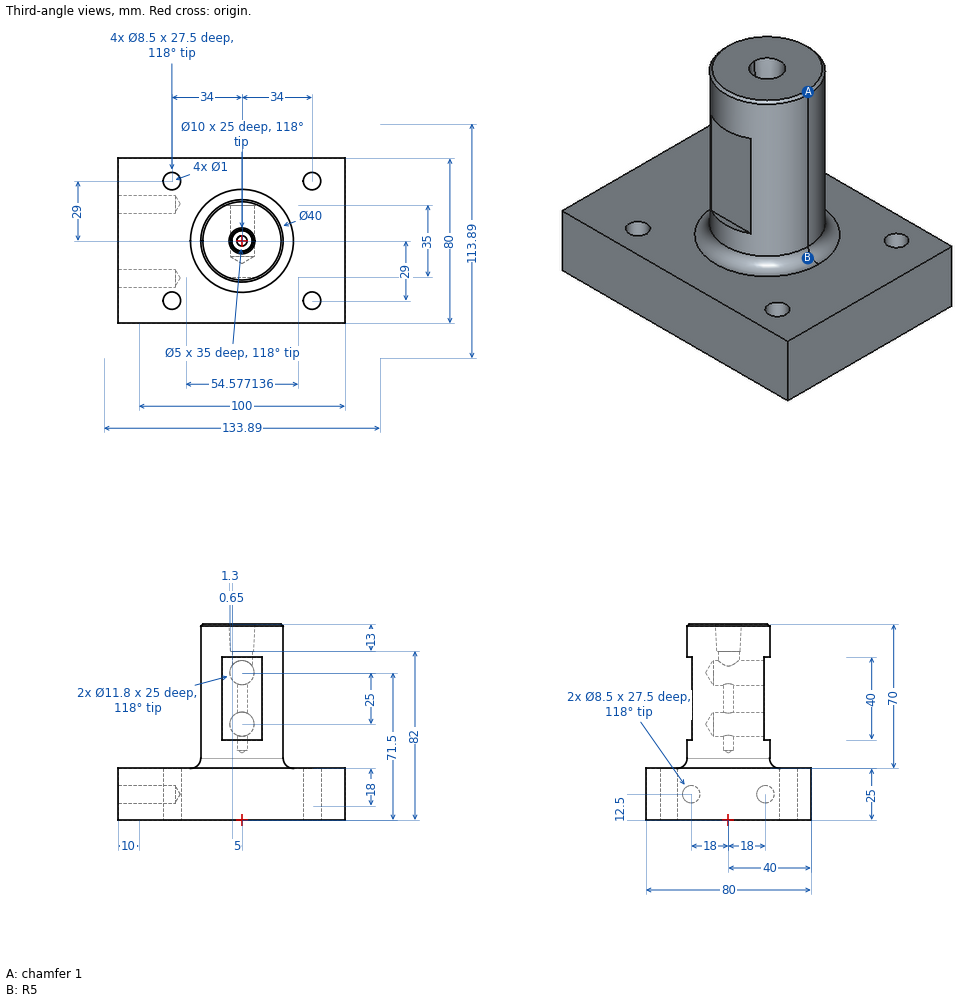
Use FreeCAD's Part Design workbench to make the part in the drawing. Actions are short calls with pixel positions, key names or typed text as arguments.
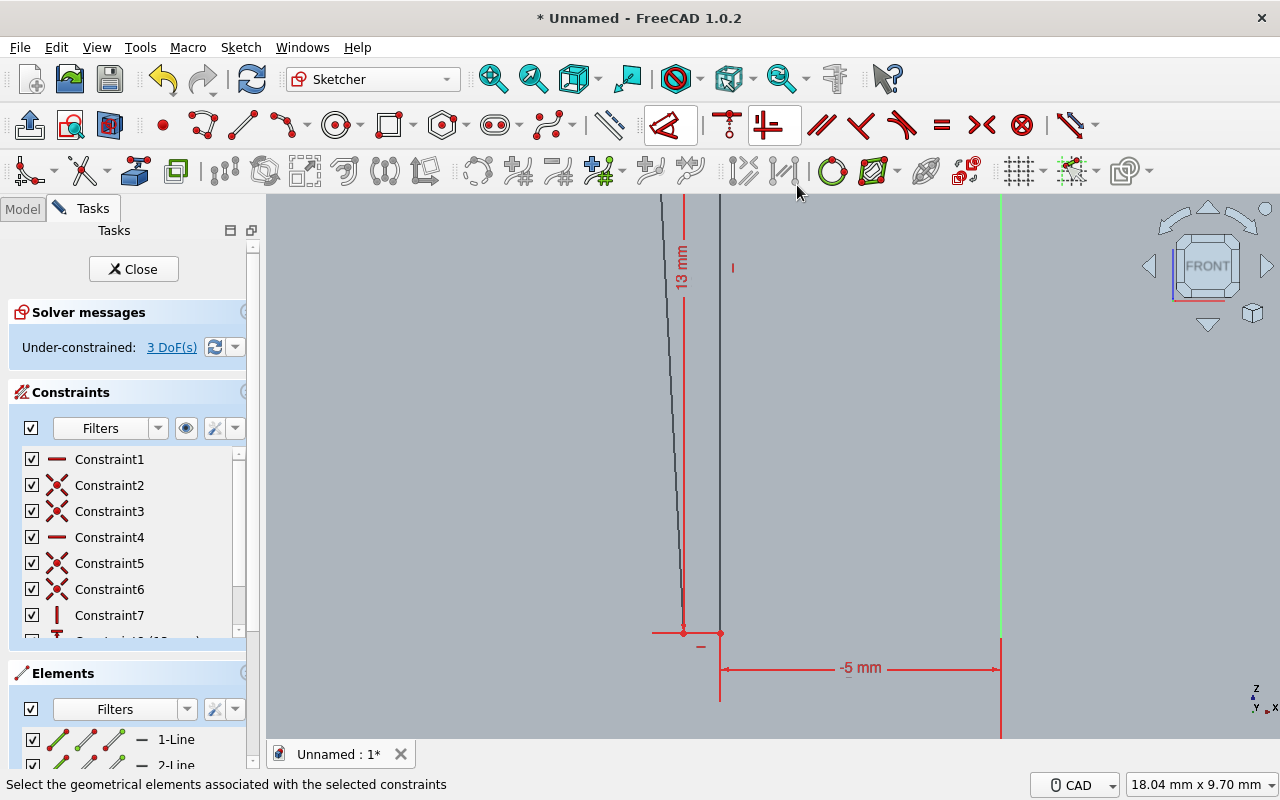
scroll(722, 630, down, 4)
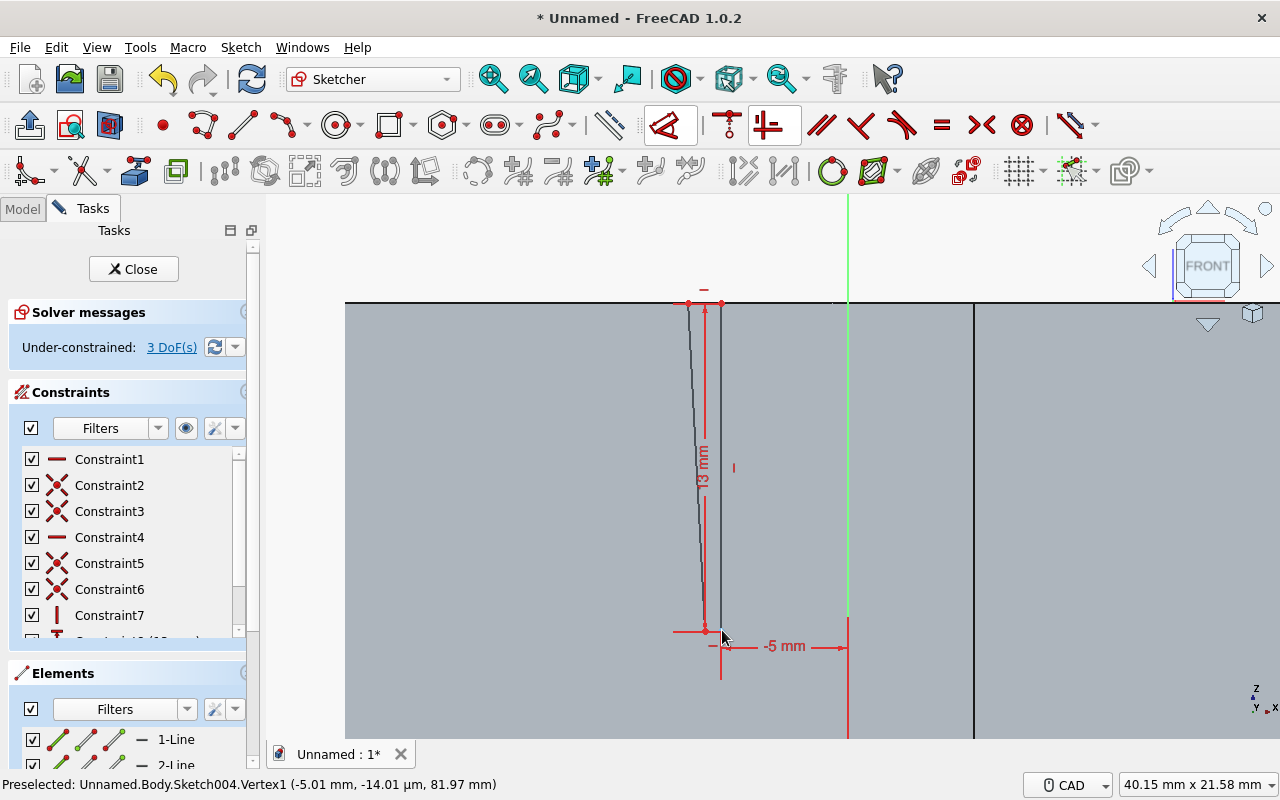
scroll(698, 304, up, 2)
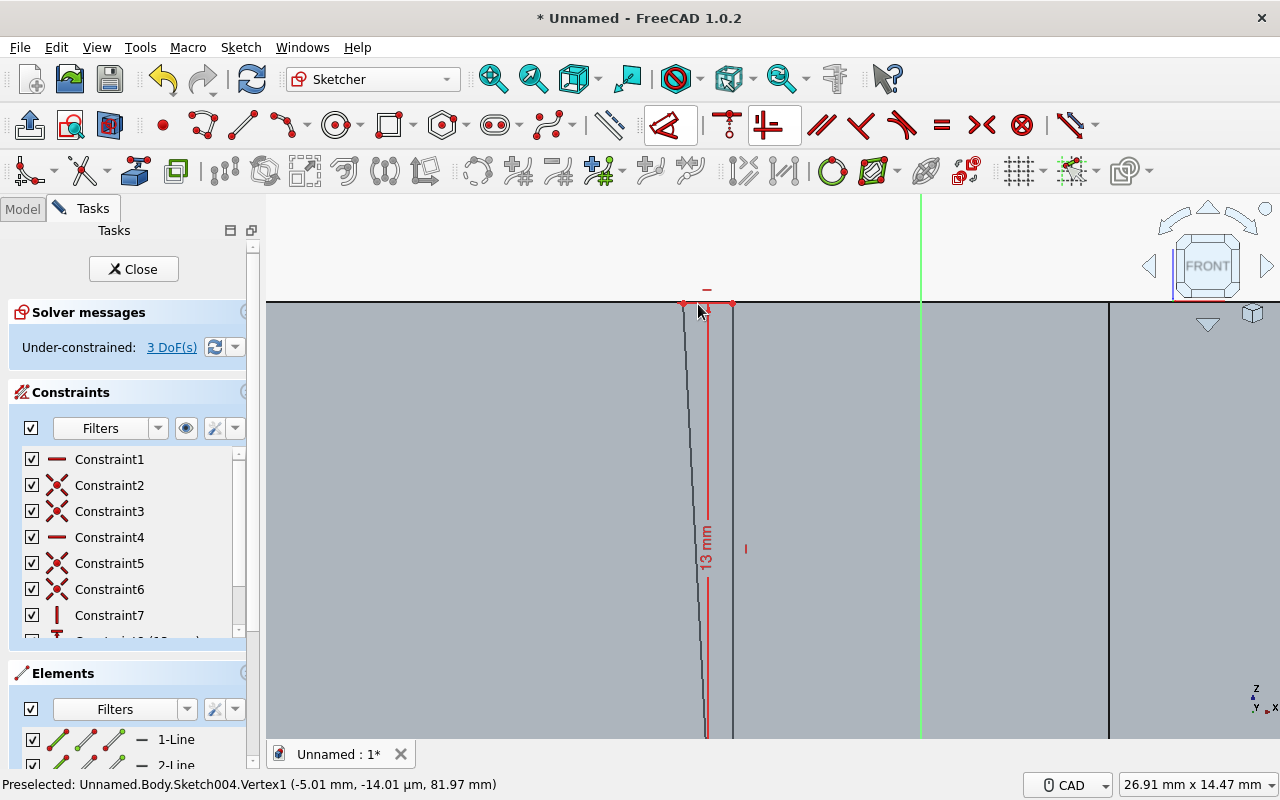
click(698, 303)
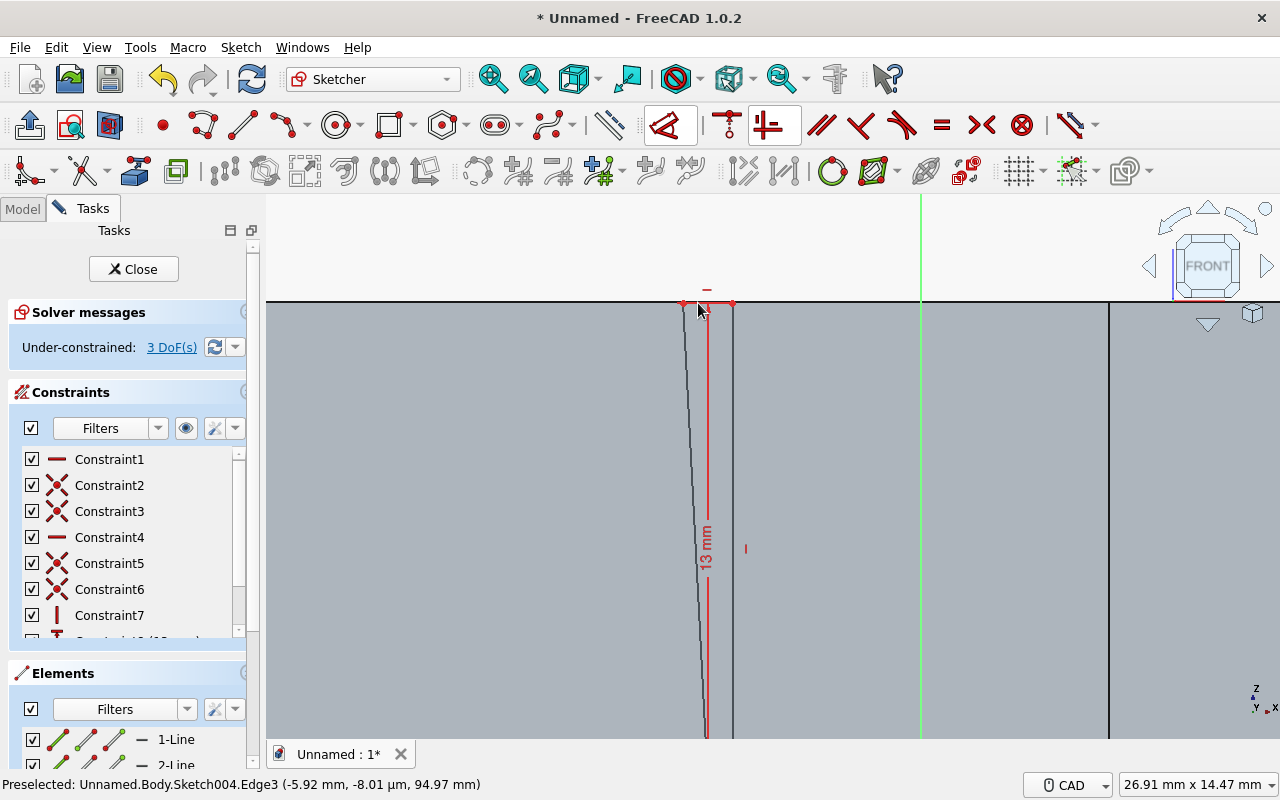
key(l)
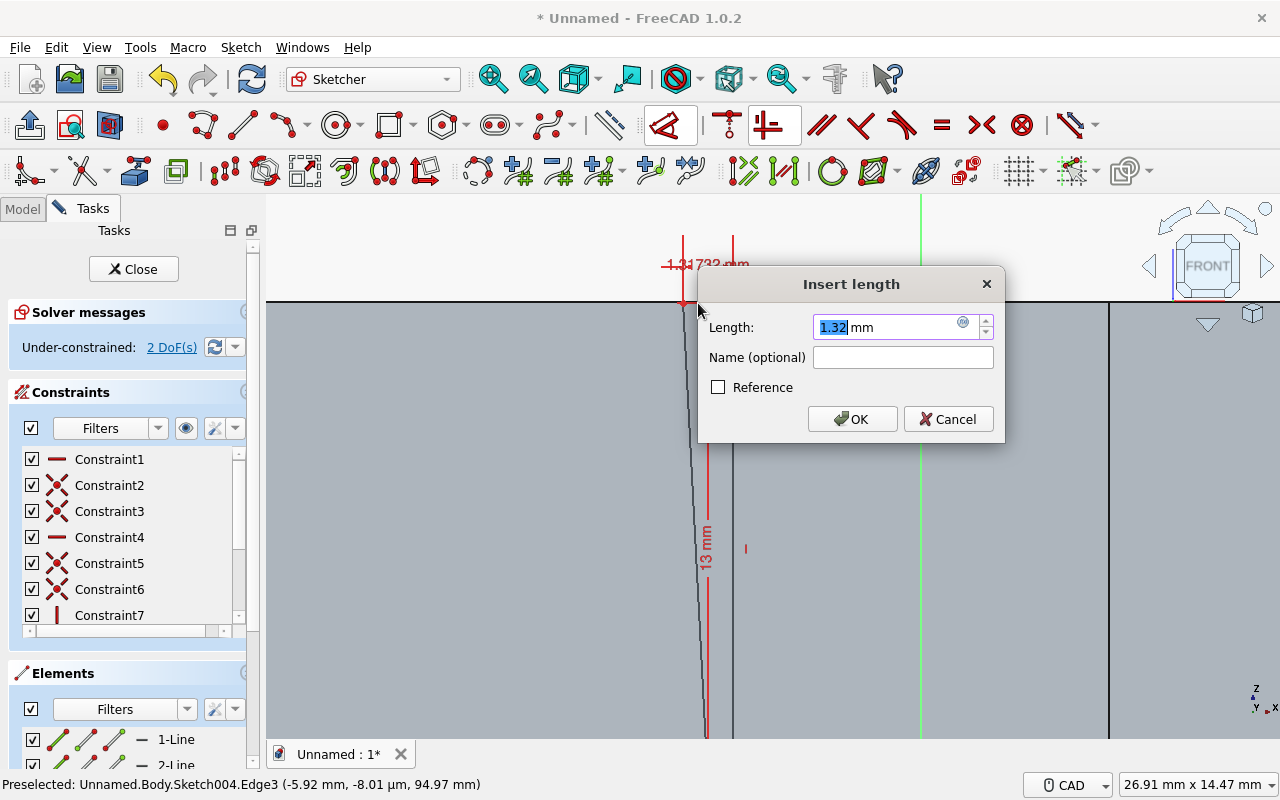
text(1.3)
key(Return)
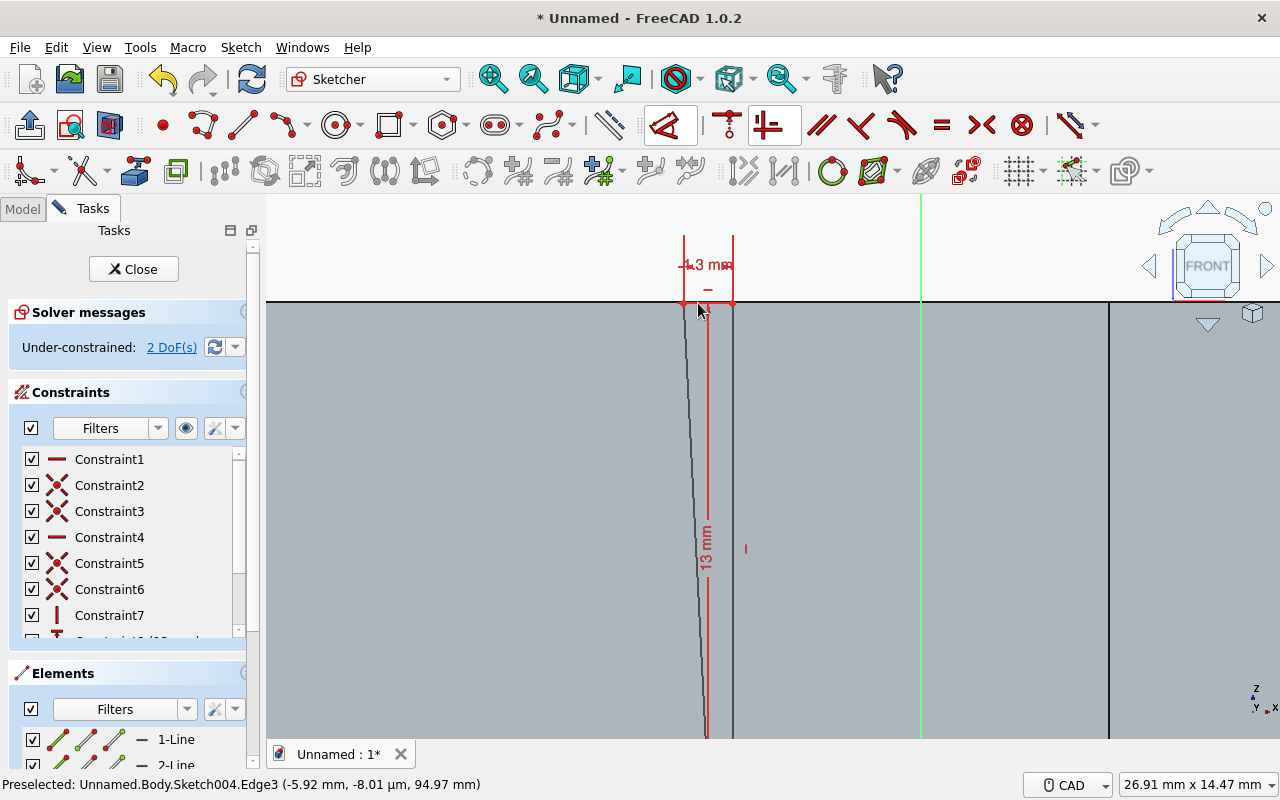
scroll(697, 303, down, 2)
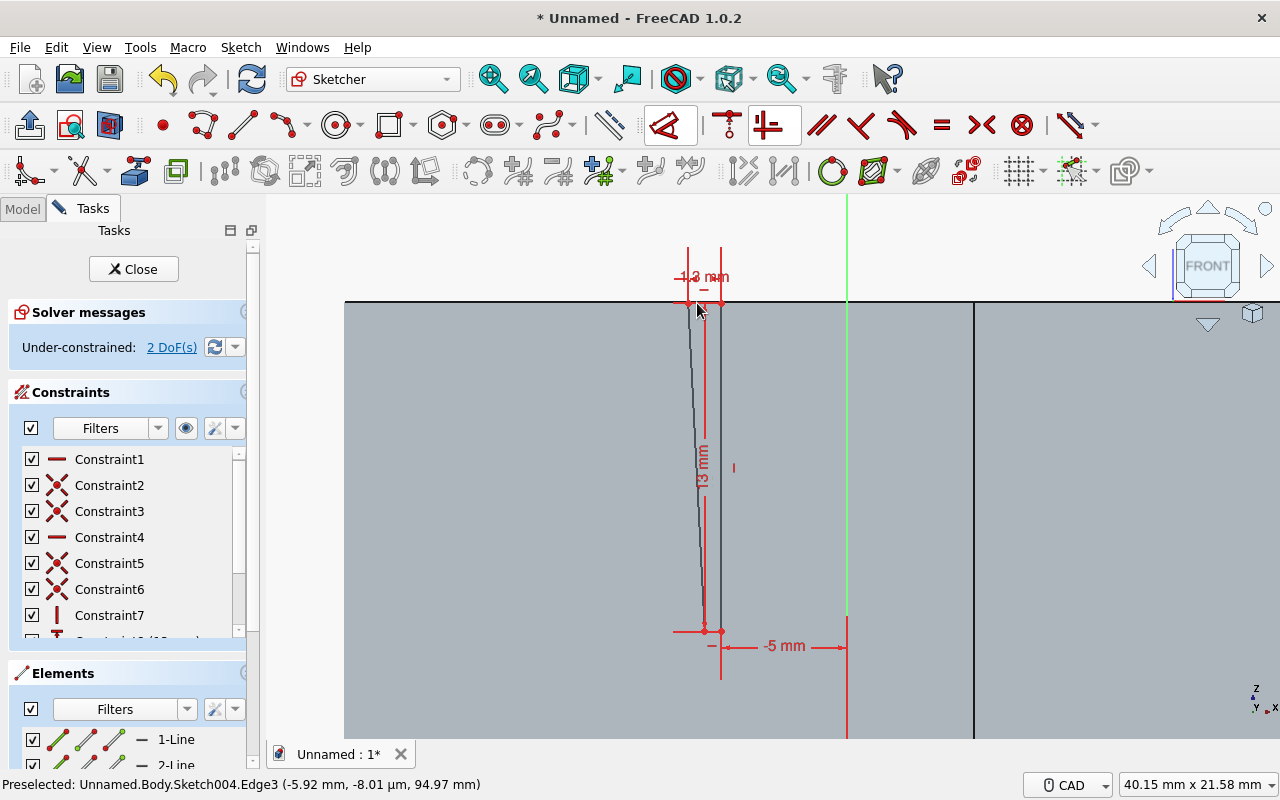
click(721, 632)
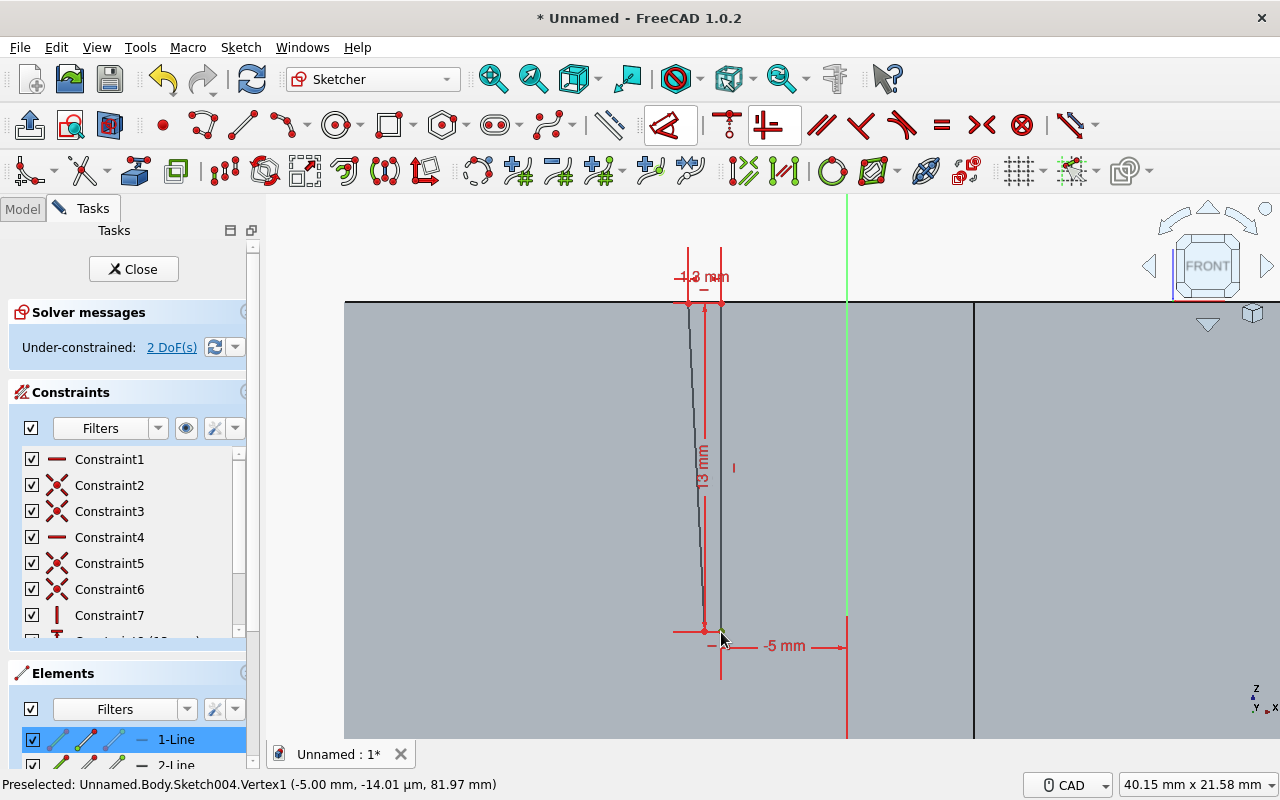
key(i)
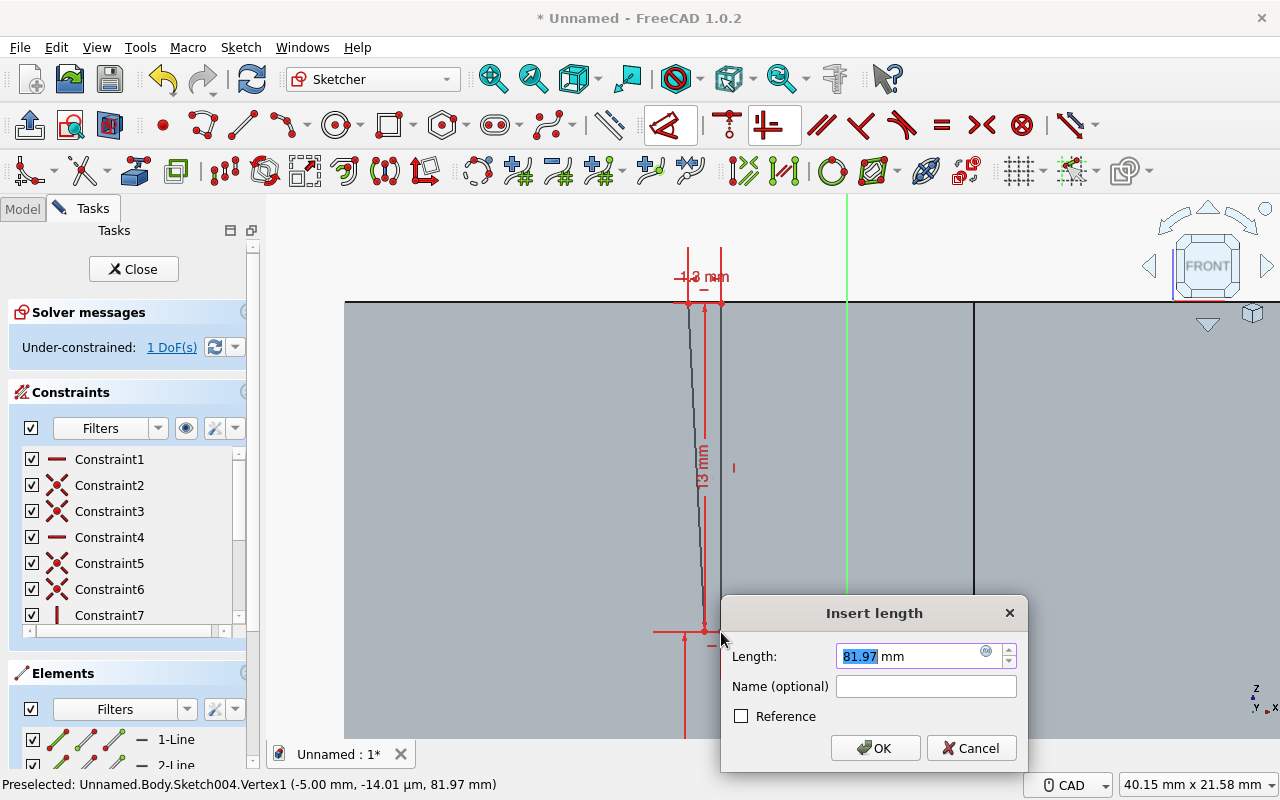
text(82)
key(Return)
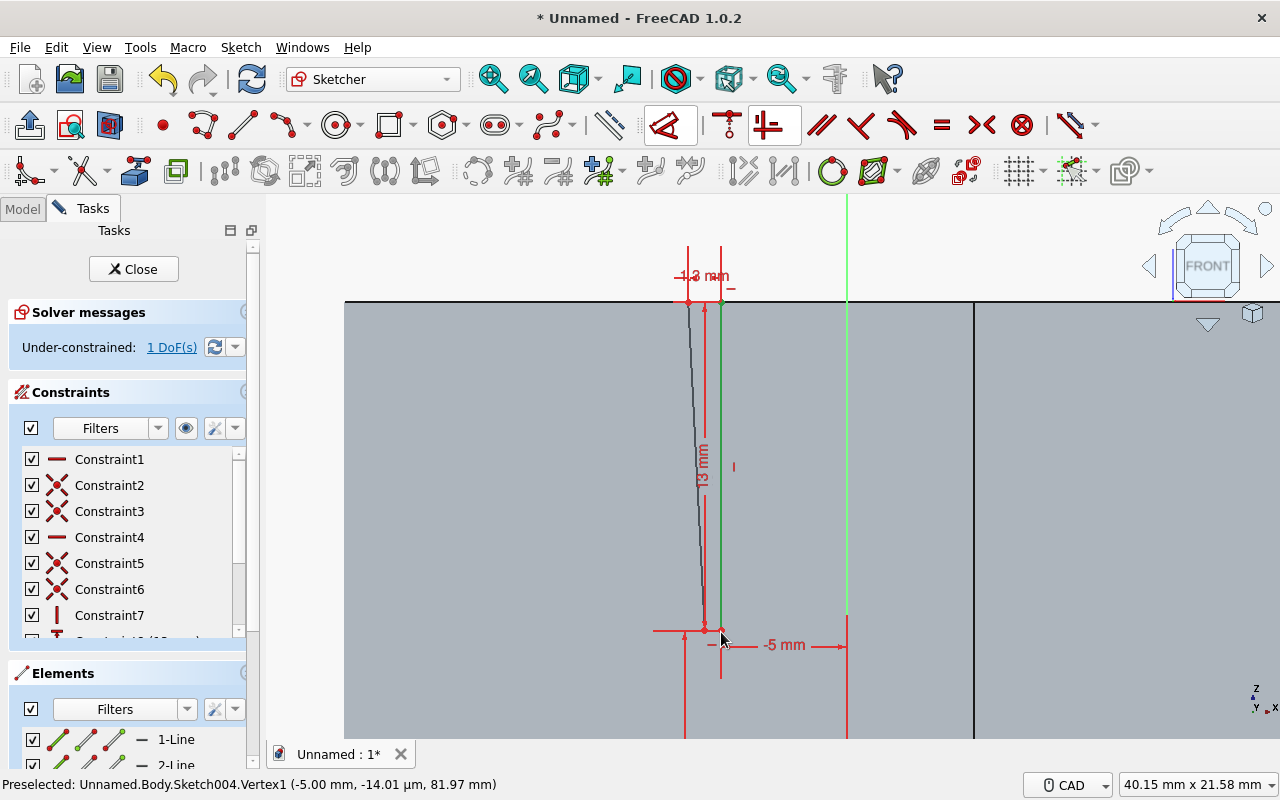
scroll(713, 631, up, 5)